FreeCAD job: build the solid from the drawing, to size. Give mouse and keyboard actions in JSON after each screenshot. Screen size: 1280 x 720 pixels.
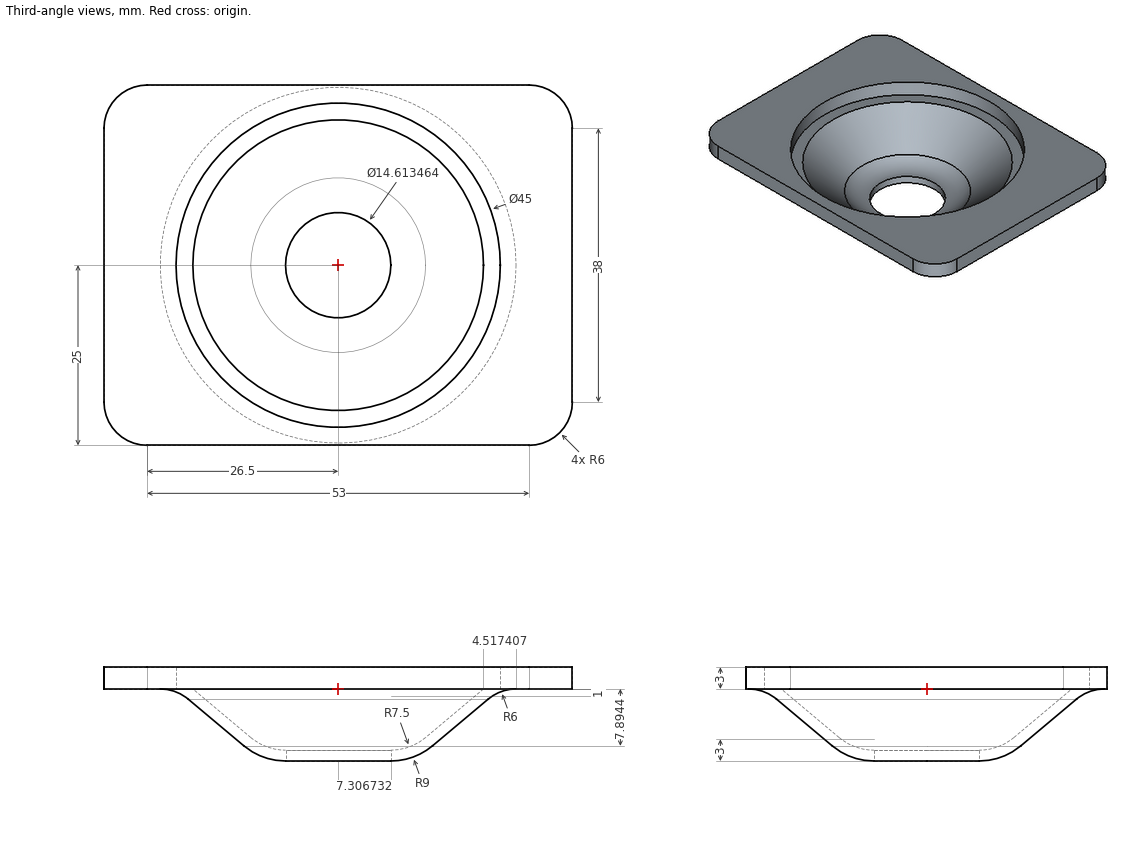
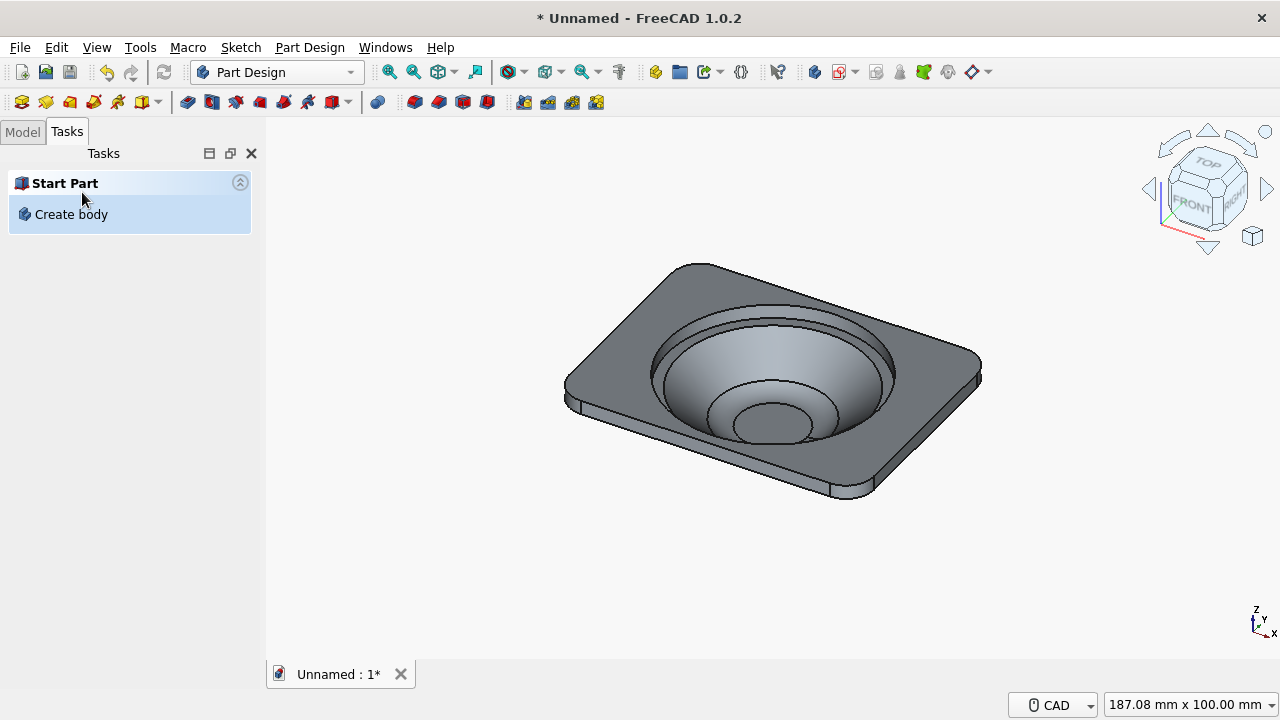
{"action": "key", "text": "5"}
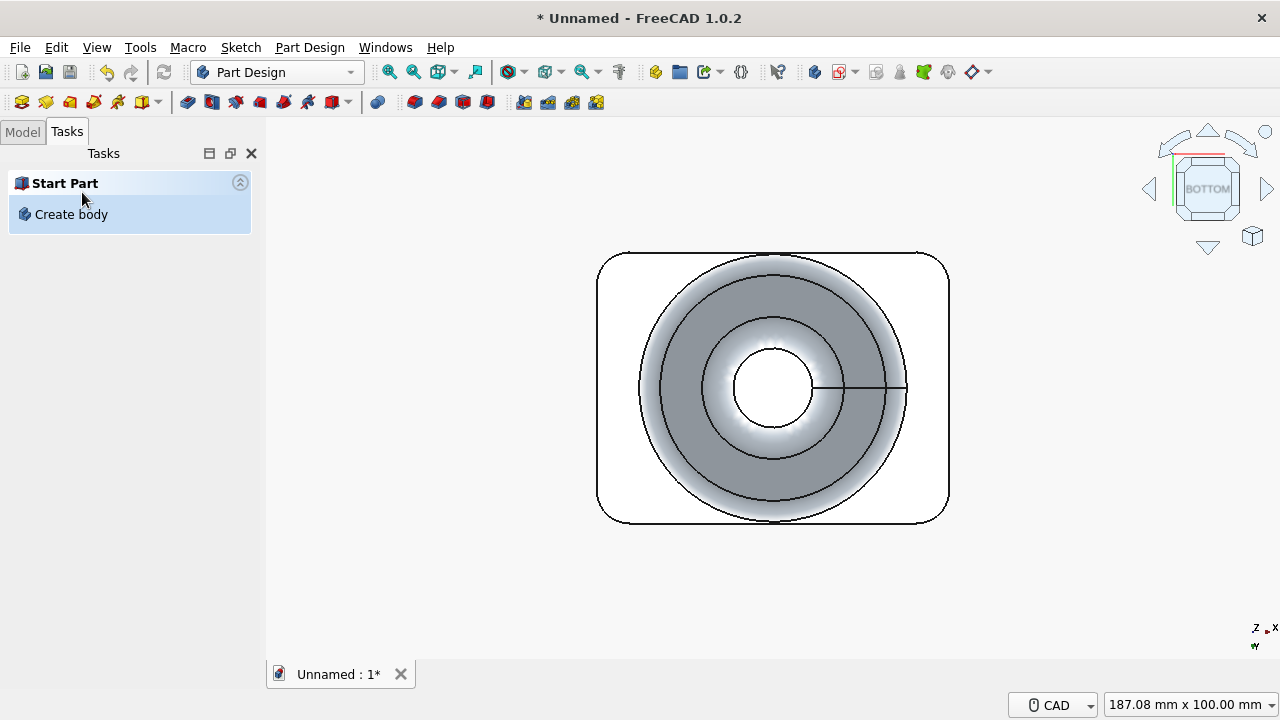
{"action": "left_click", "coordinate": [773, 387]}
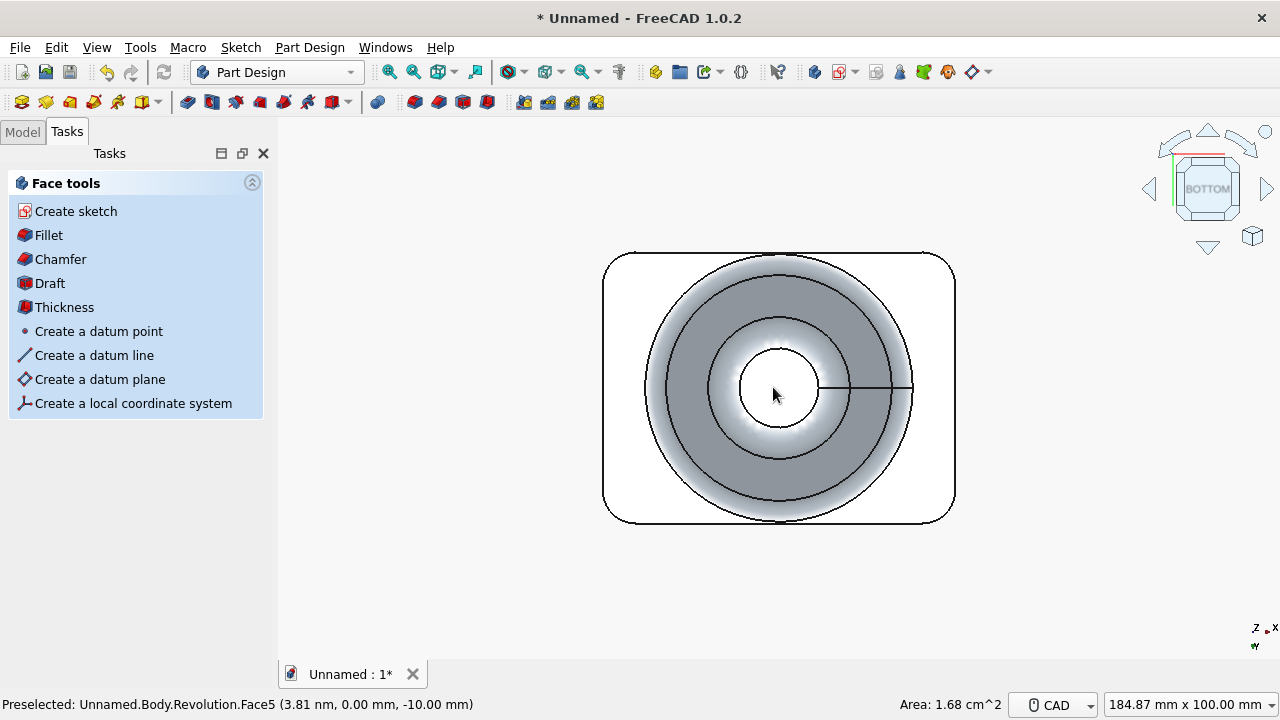
{"action": "left_click", "coordinate": [840, 72]}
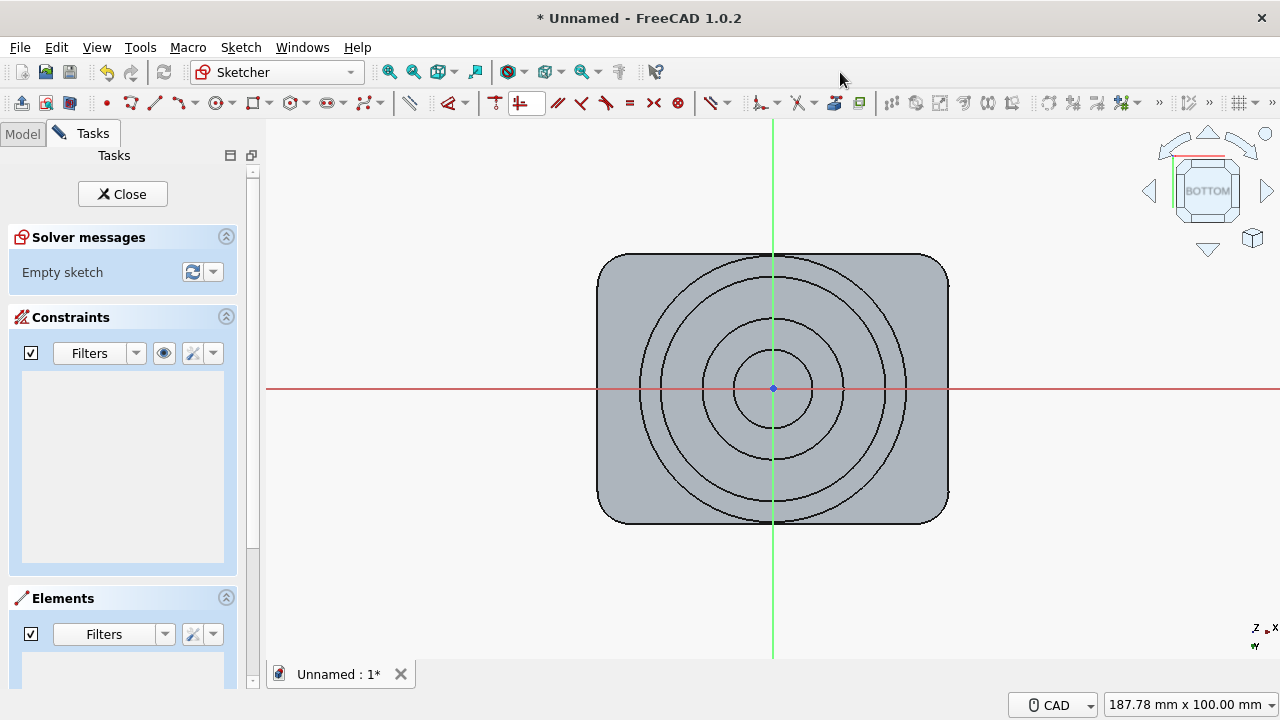
{"action": "scroll", "coordinate": [795, 389], "scroll_direction": "up", "scroll_amount": 7}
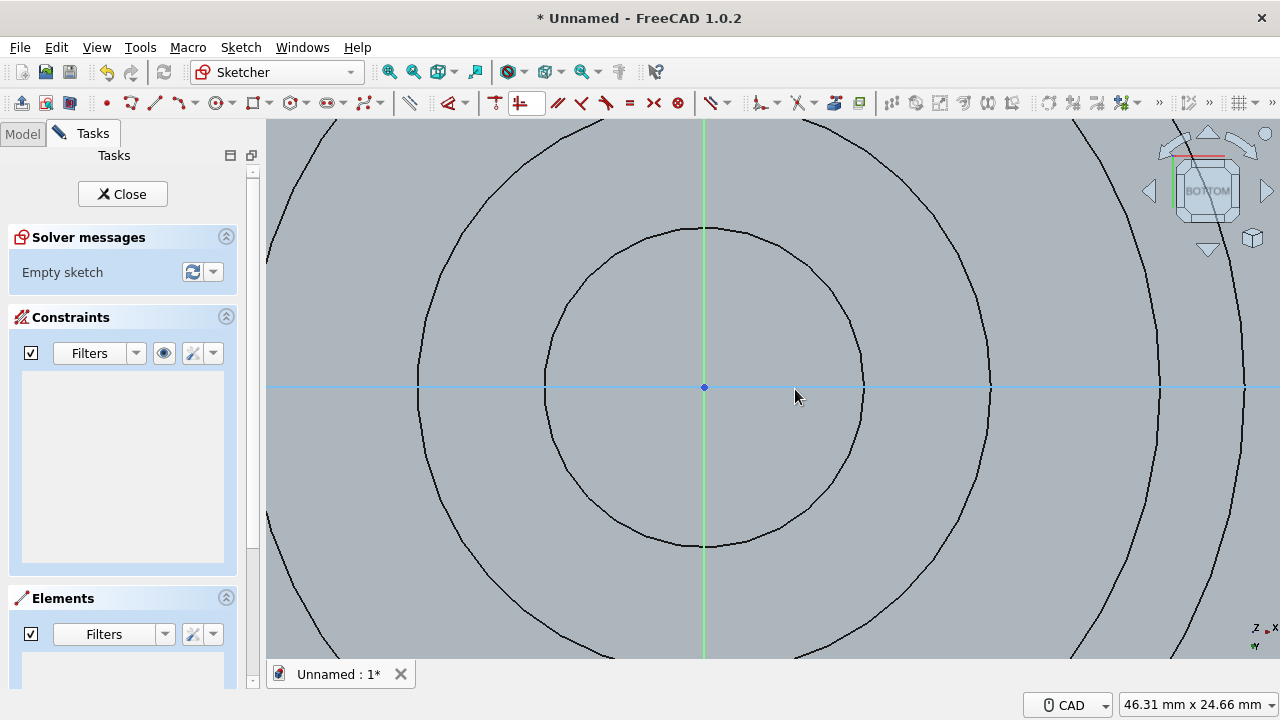
{"action": "left_click", "coordinate": [216, 104]}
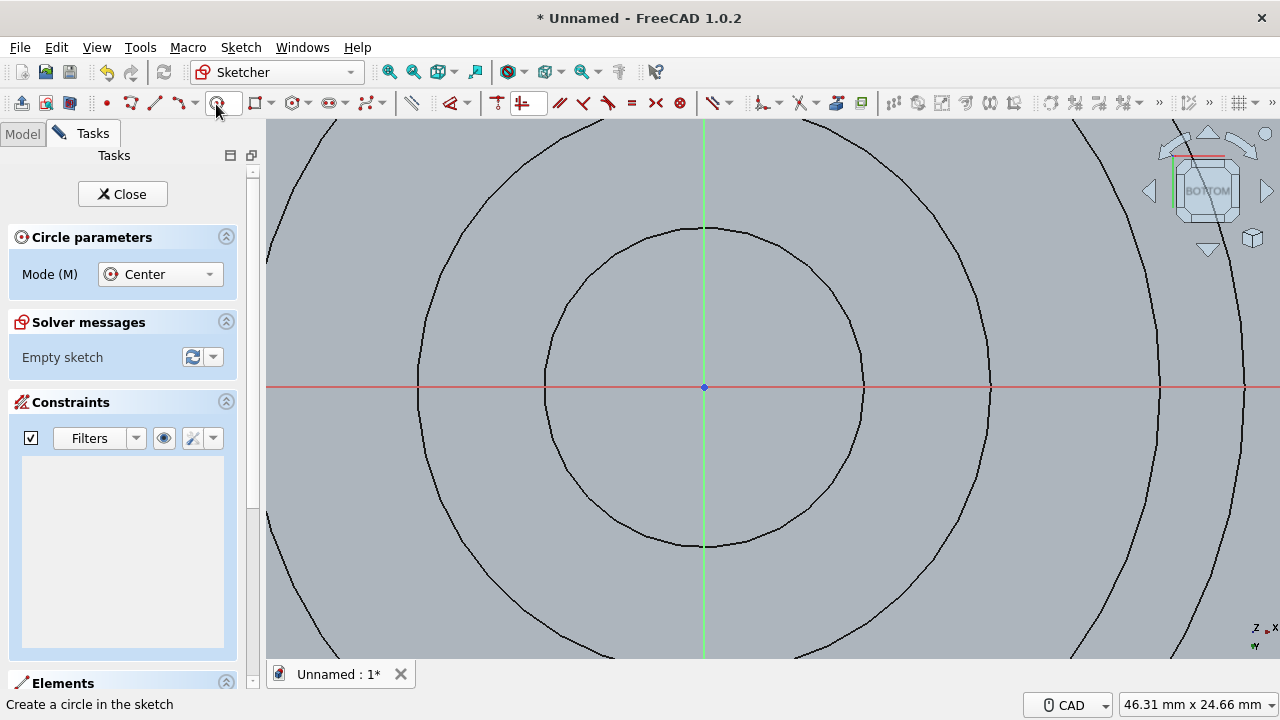
{"action": "left_click", "coordinate": [704, 387]}
{"action": "mouse_move", "coordinate": [817, 274]}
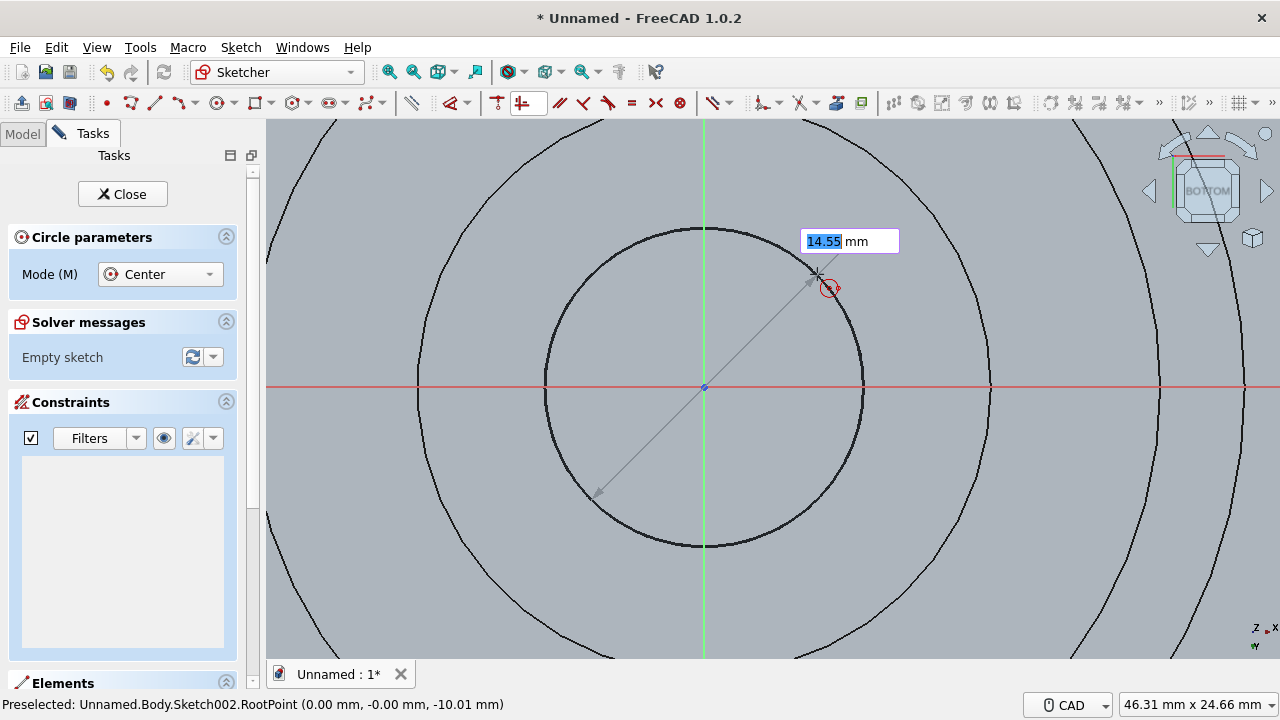
{"action": "type", "text": "14.613464"}
{"action": "key", "text": "Return"}
{"action": "key", "text": "Escape"}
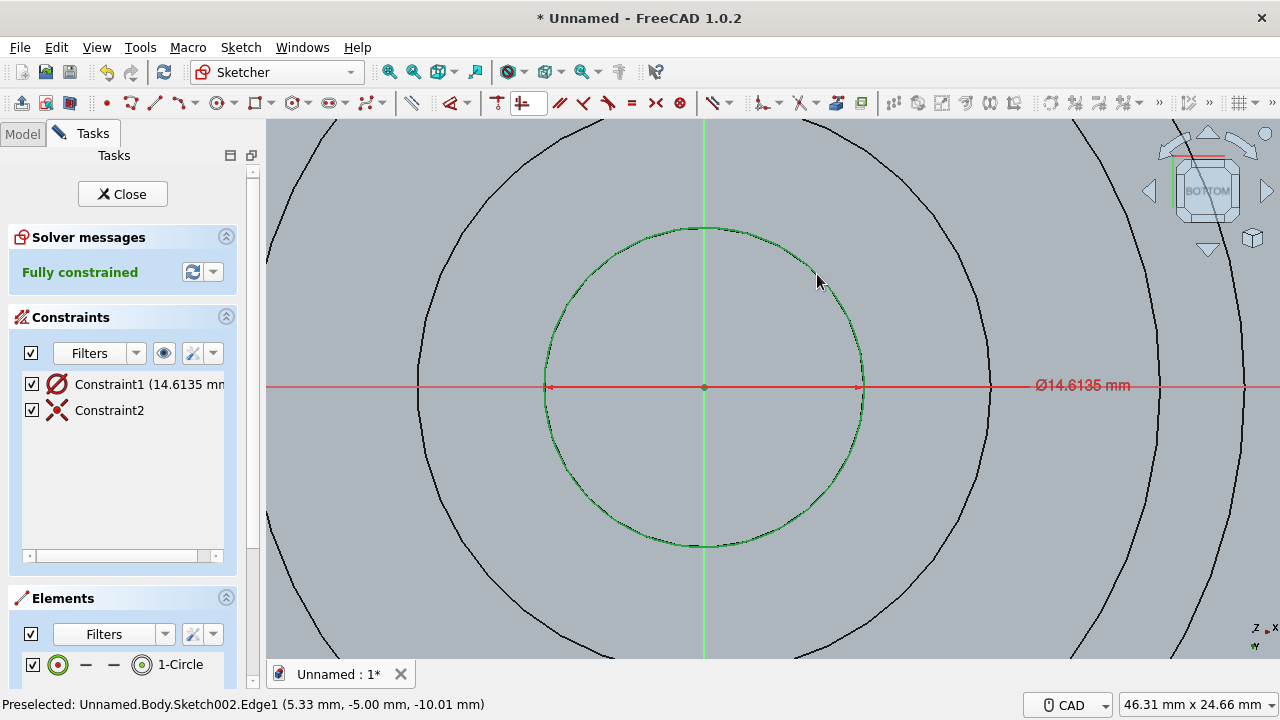
{"action": "left_click", "coordinate": [123, 194]}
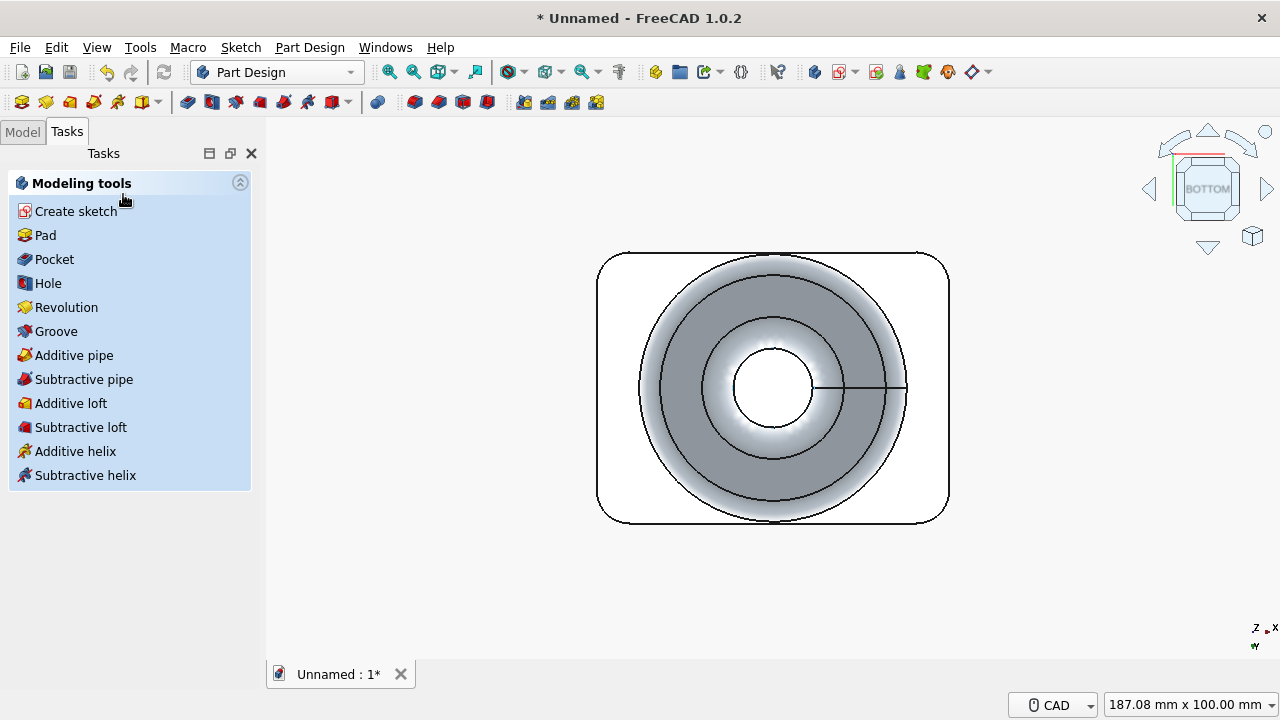
{"action": "left_click", "coordinate": [188, 102]}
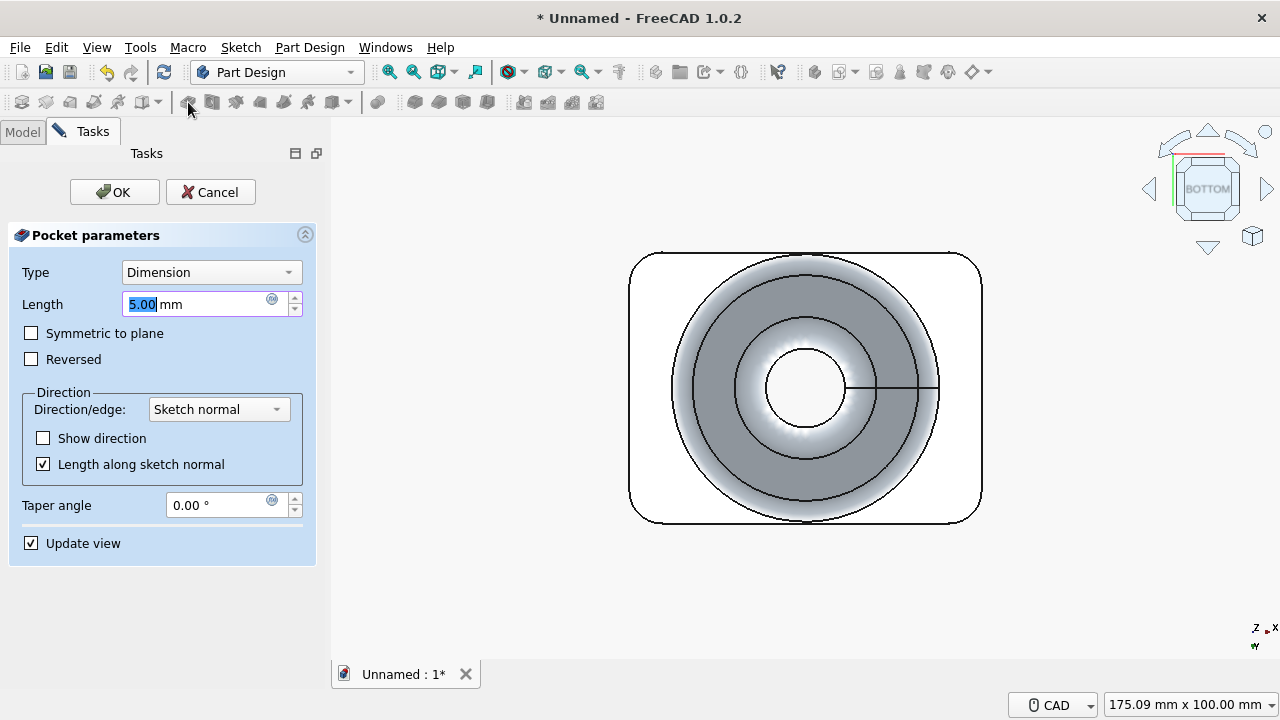
{"action": "type", "text": "3"}
{"action": "key", "text": "Tab"}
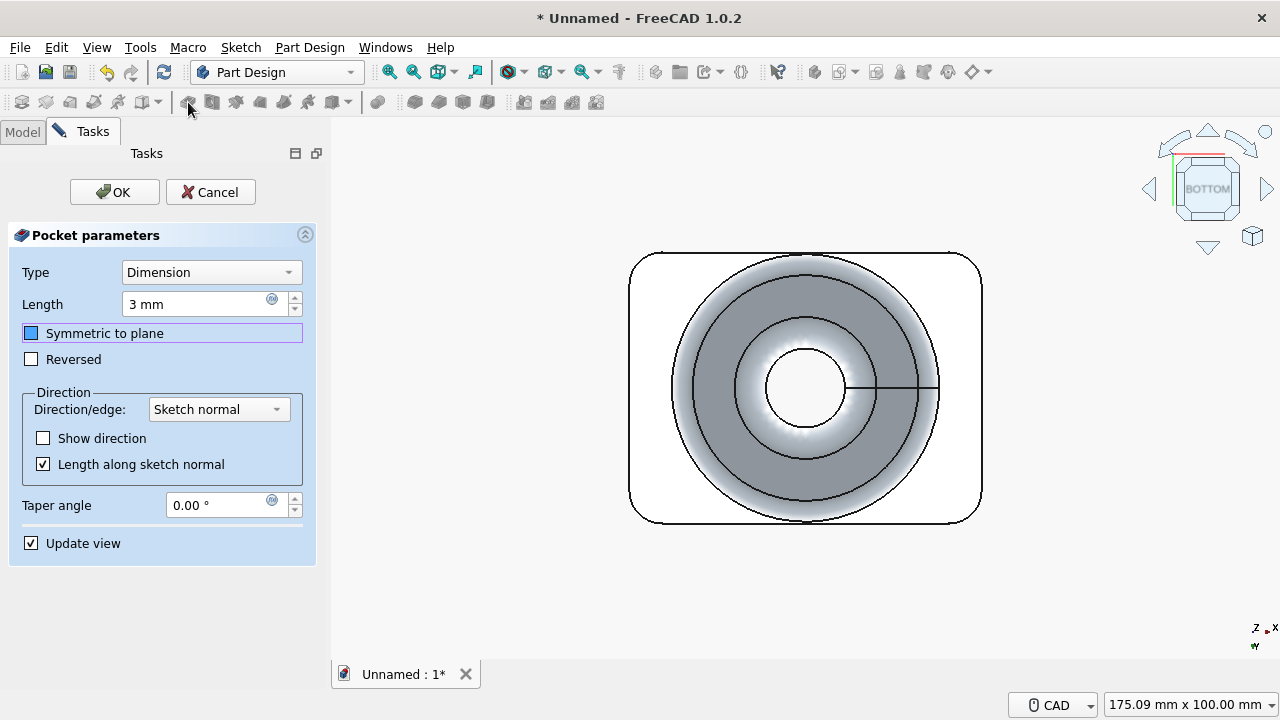
{"action": "left_click", "coordinate": [115, 192]}